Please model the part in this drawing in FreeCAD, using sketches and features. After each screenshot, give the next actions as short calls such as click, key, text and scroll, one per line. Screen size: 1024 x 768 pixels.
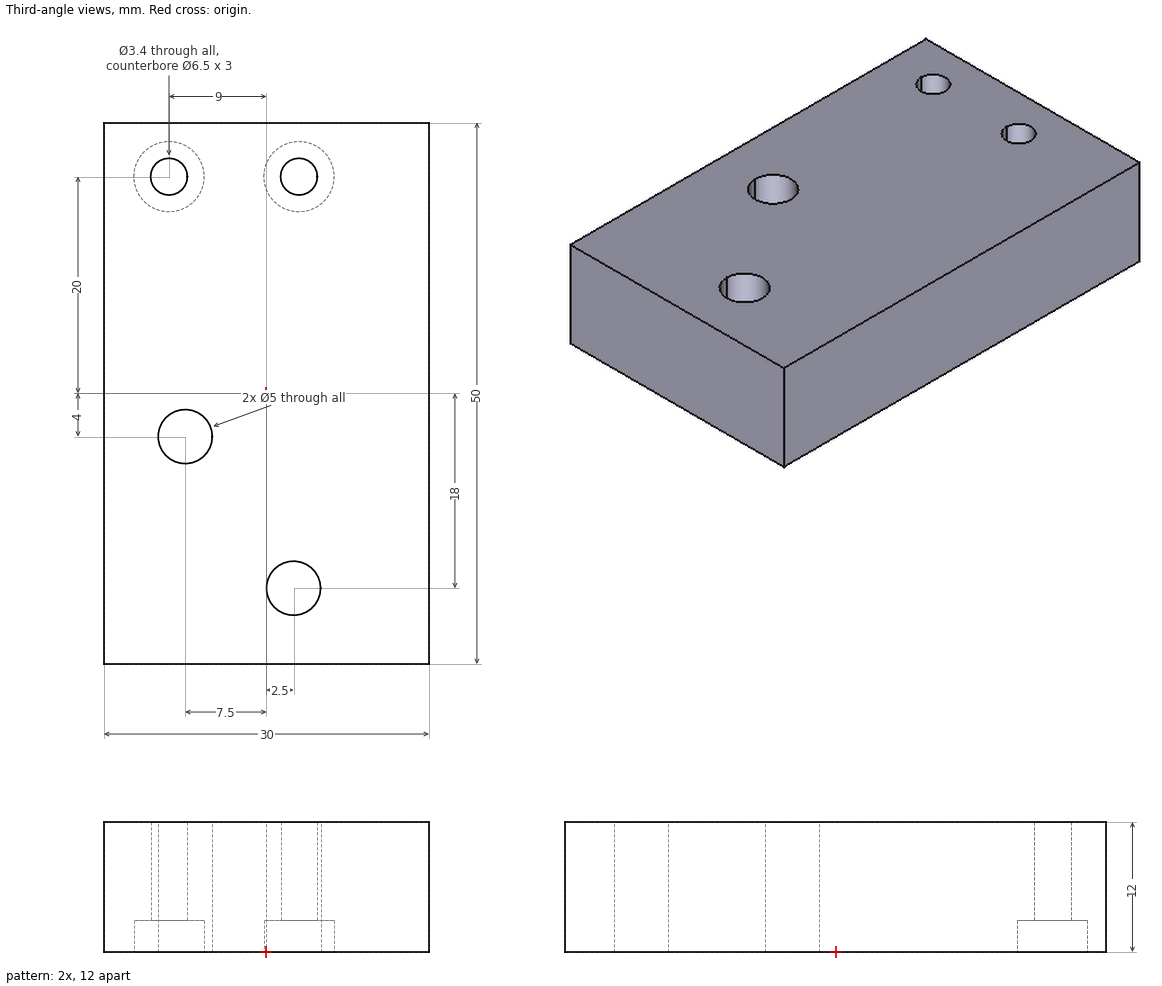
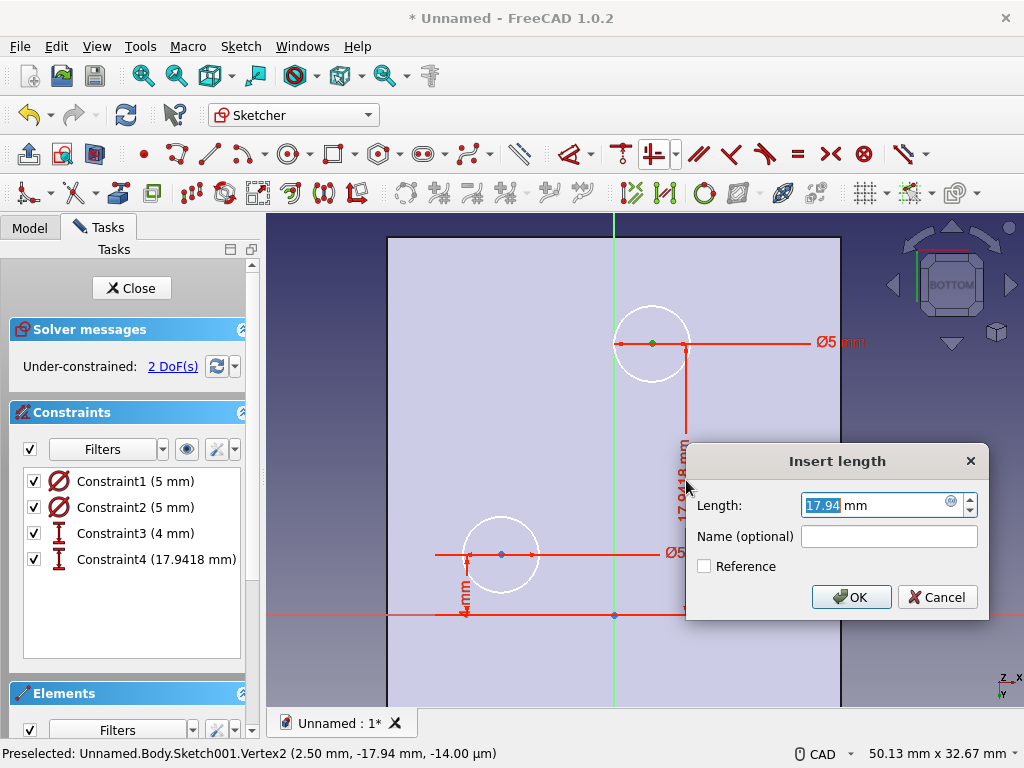
text(18)
key(Return)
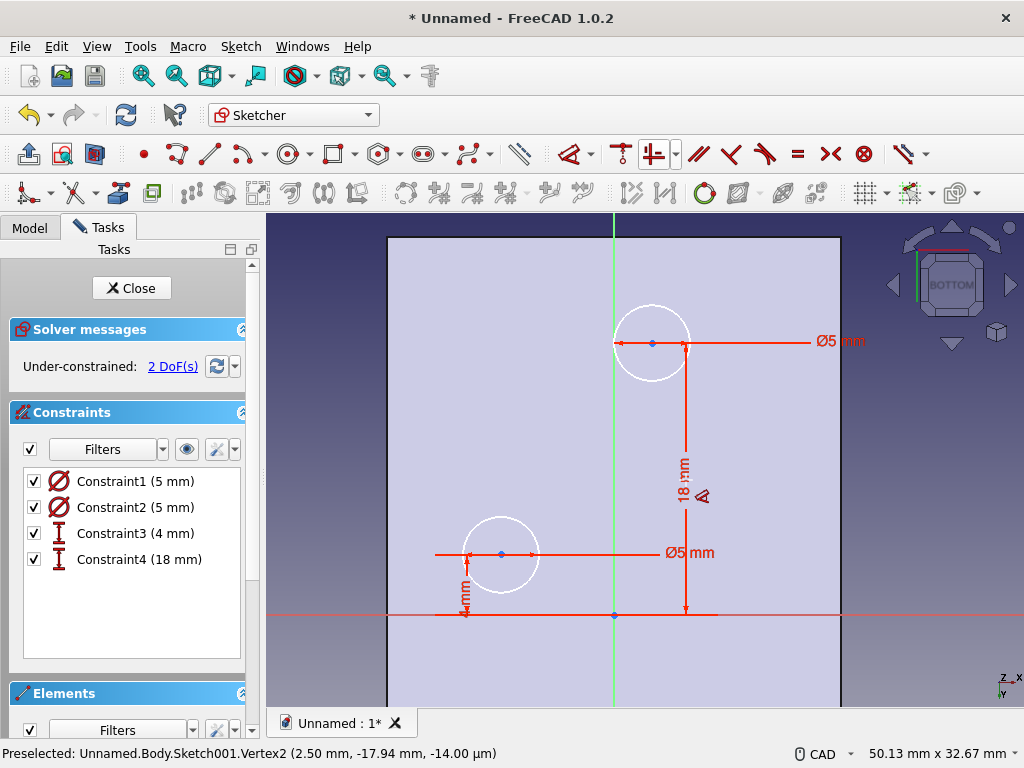
click(501, 555)
click(558, 649)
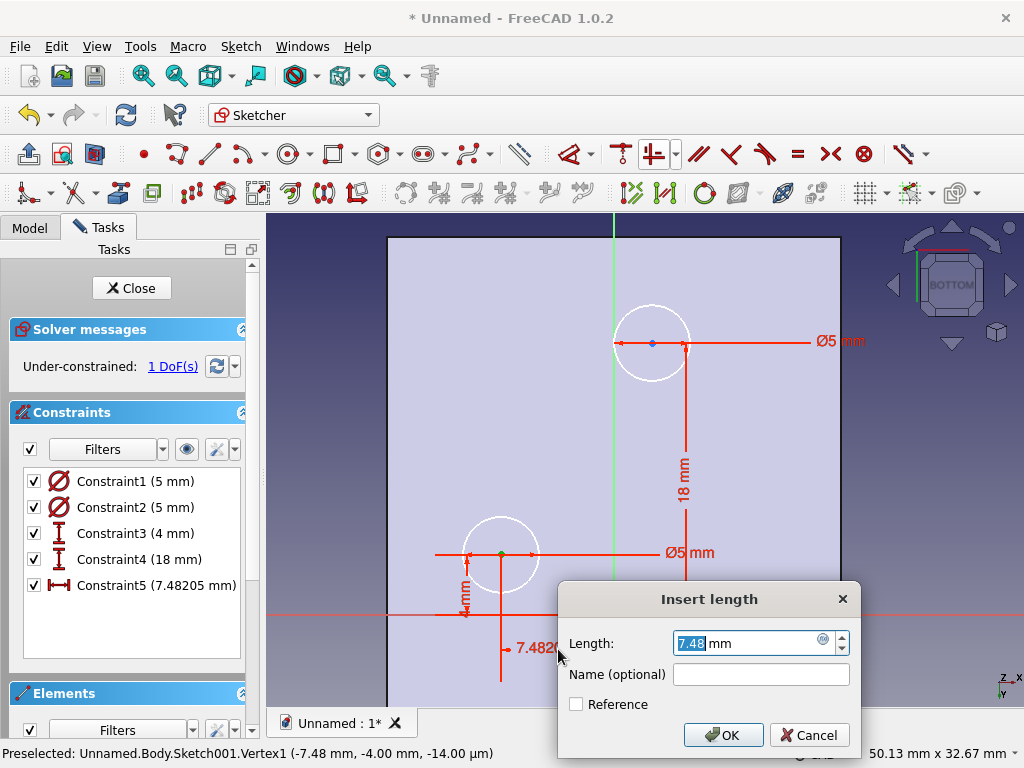
text(7.5)
key(Return)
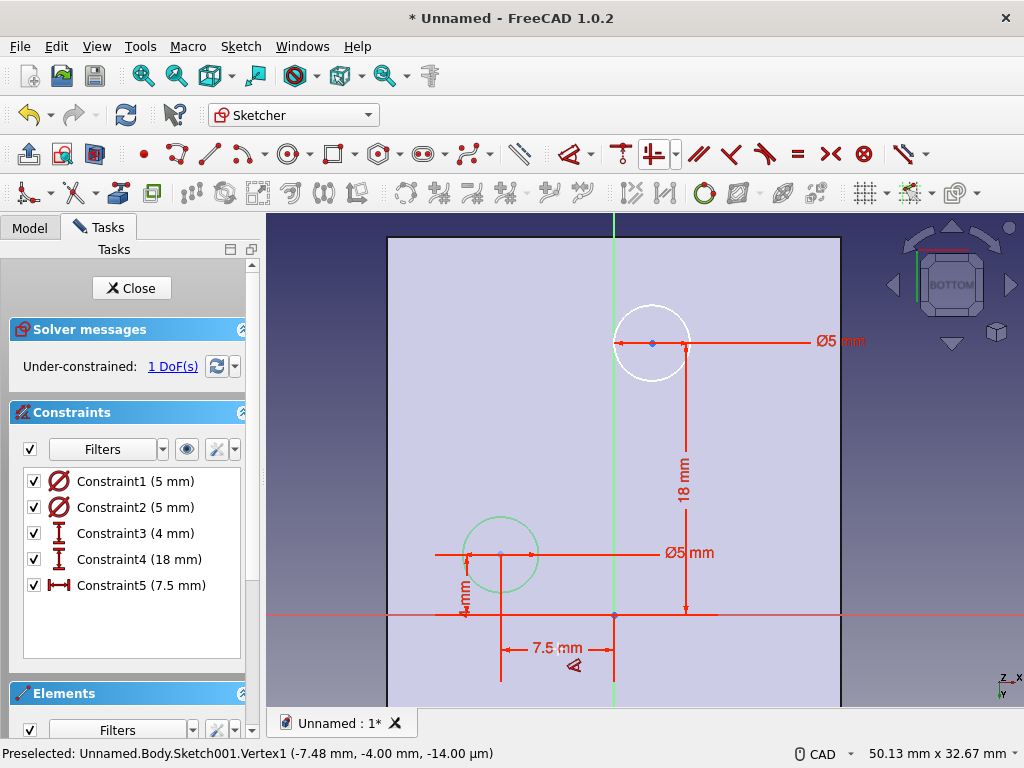
click(652, 343)
click(633, 649)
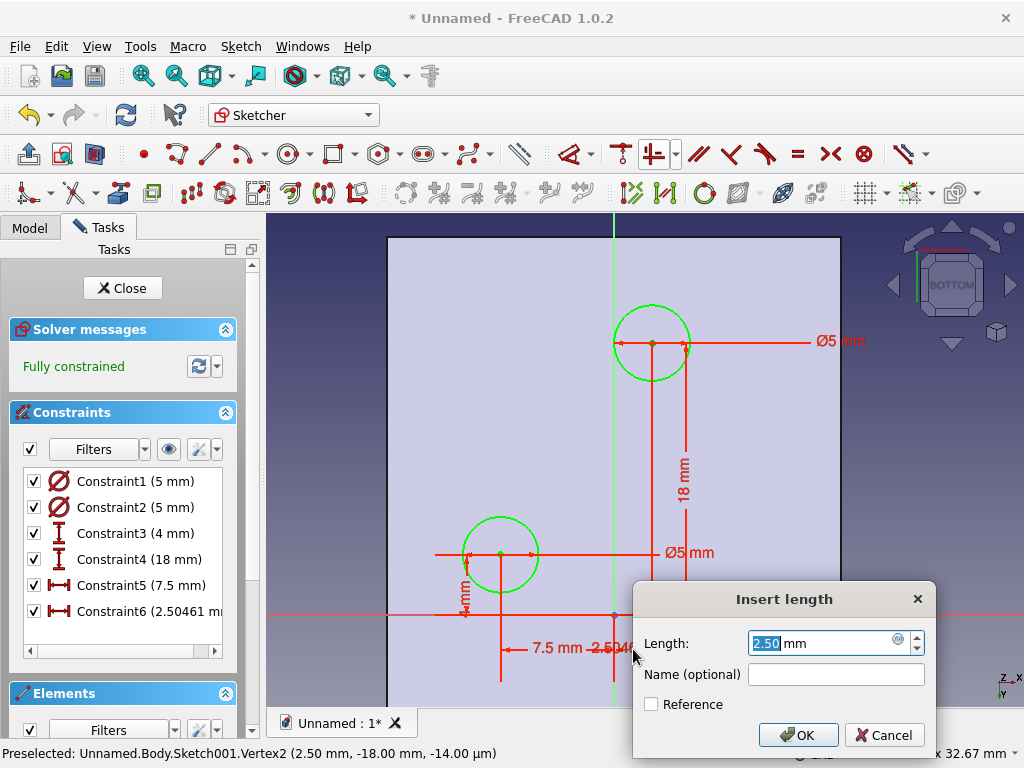
text(2.5)
key(Return)
key(Escape)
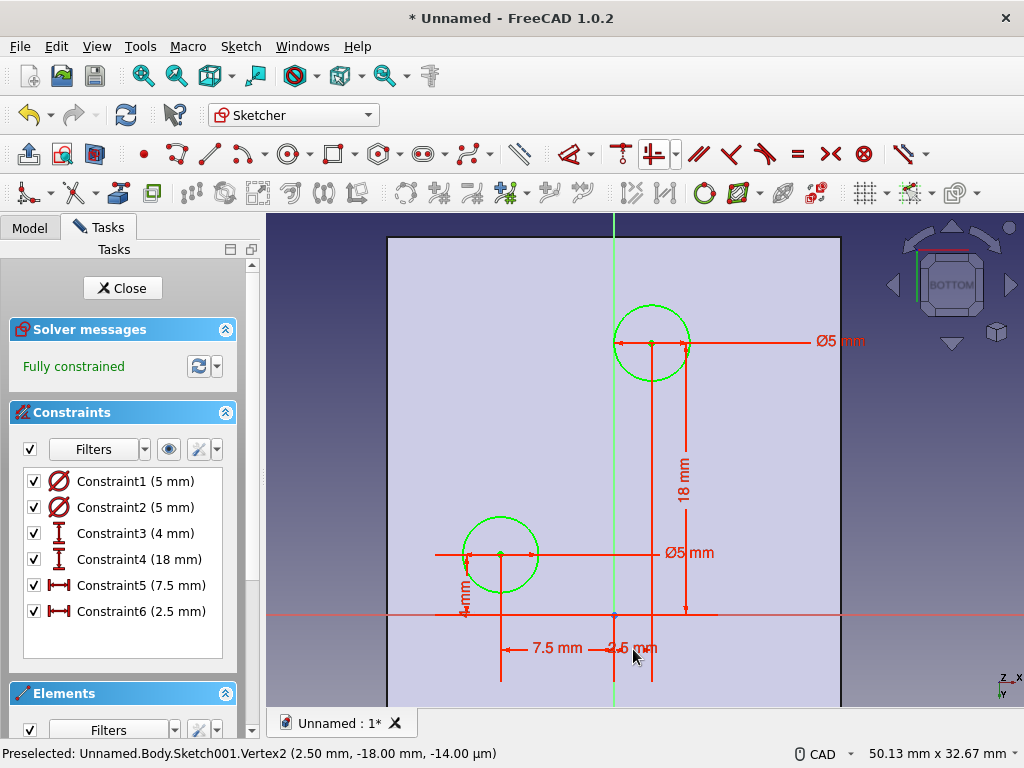
click(123, 288)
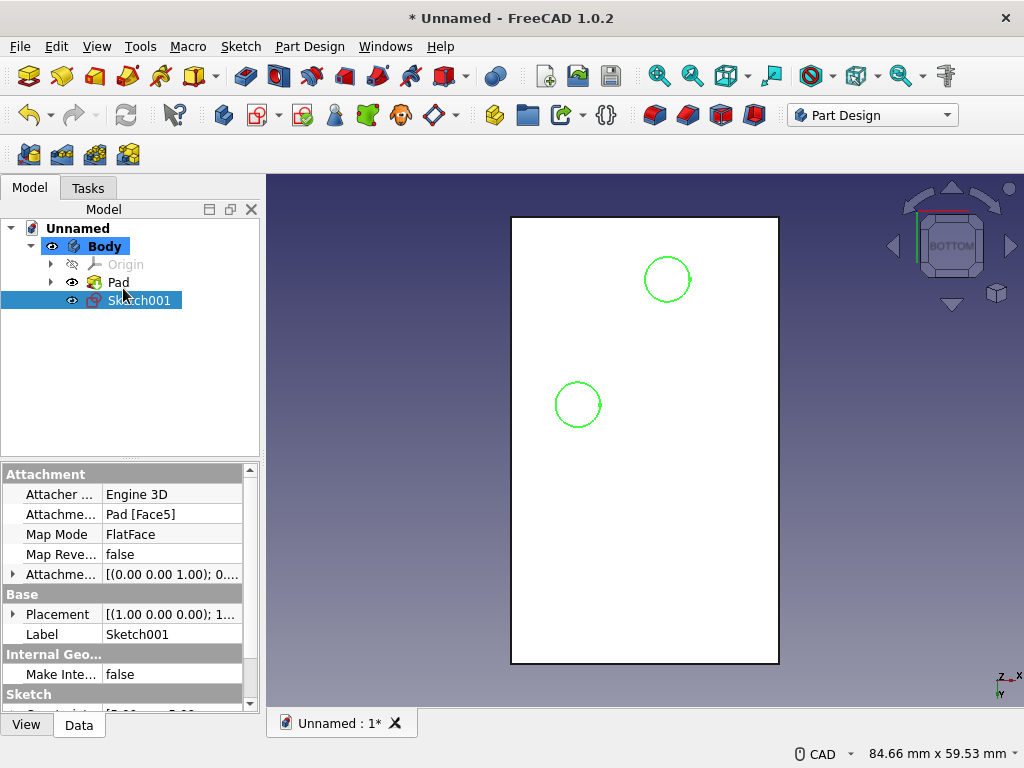
click(279, 76)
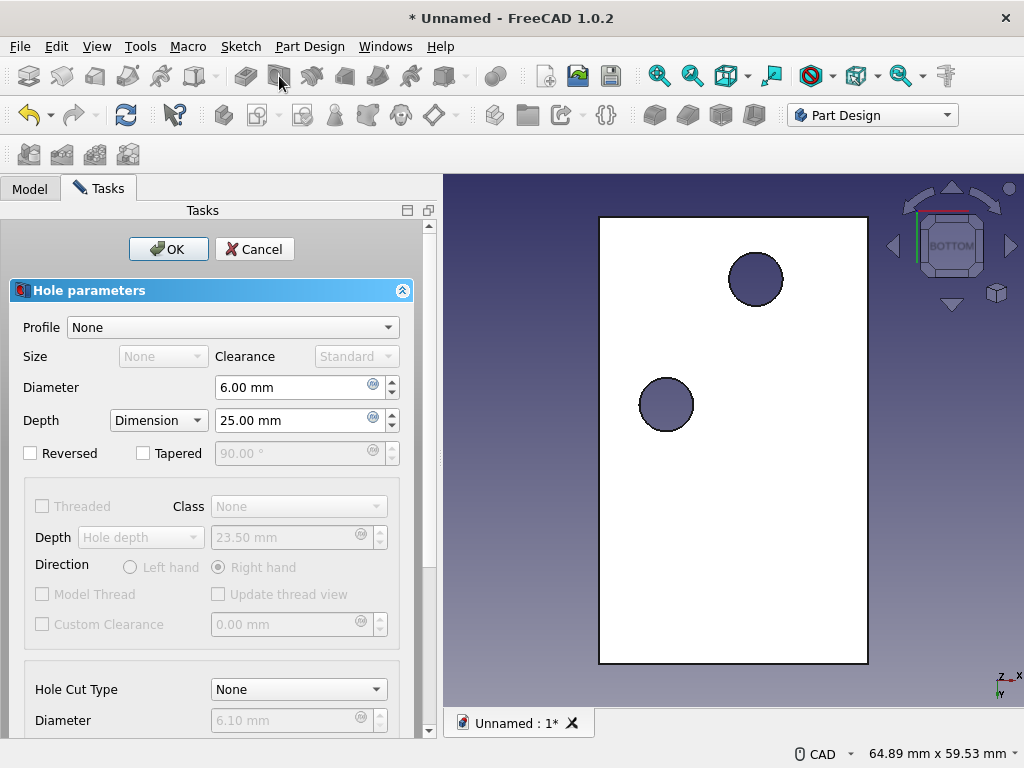
triple_click(300, 388)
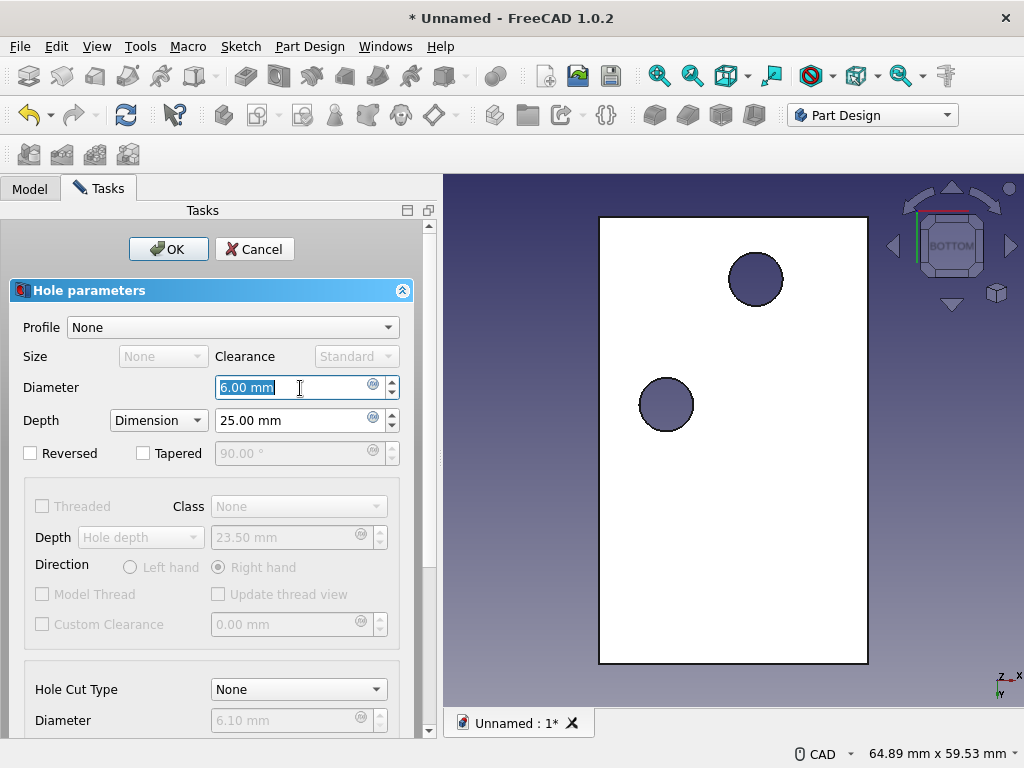
text(5)
key(Tab)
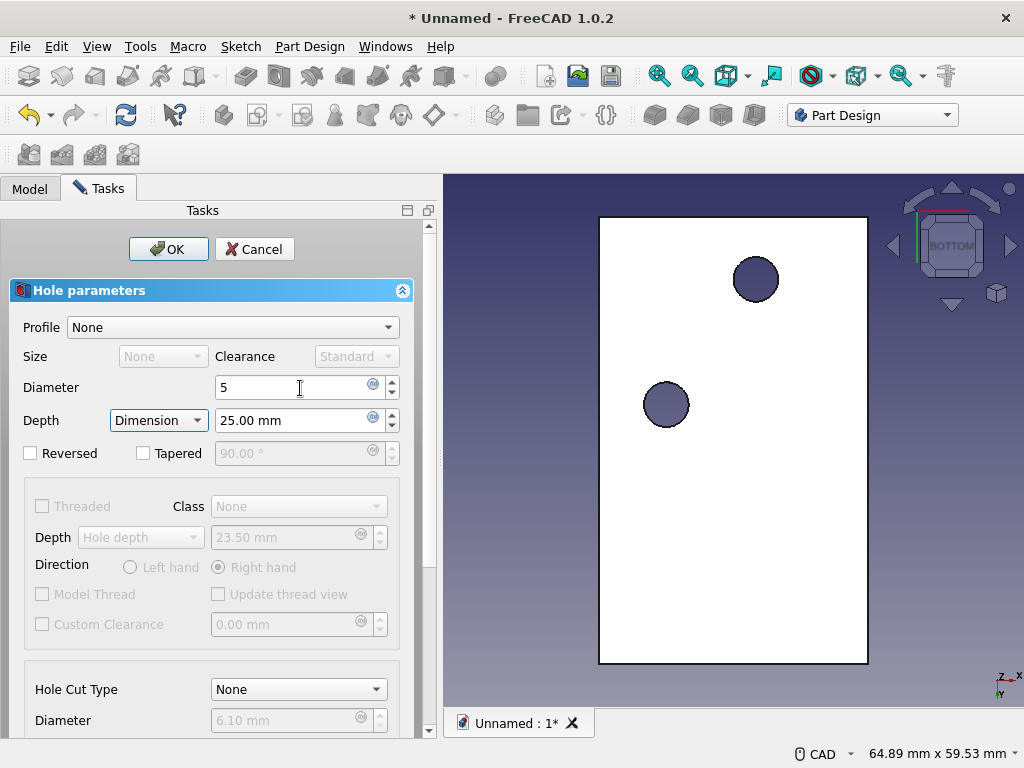
click(160, 420)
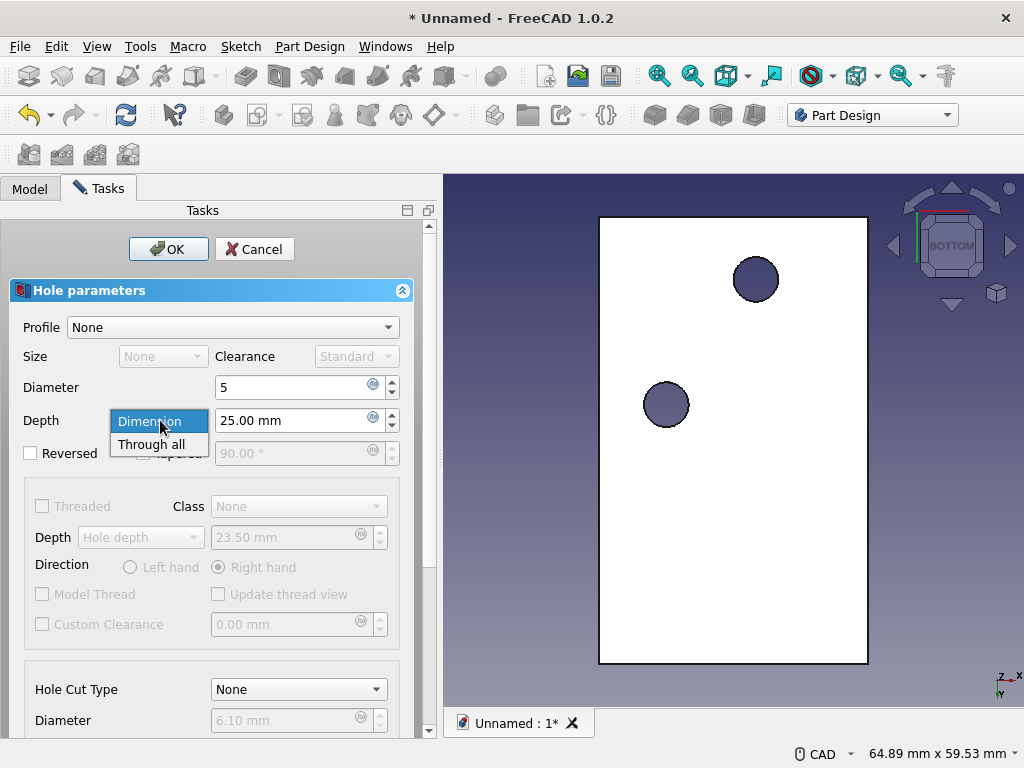
click(158, 444)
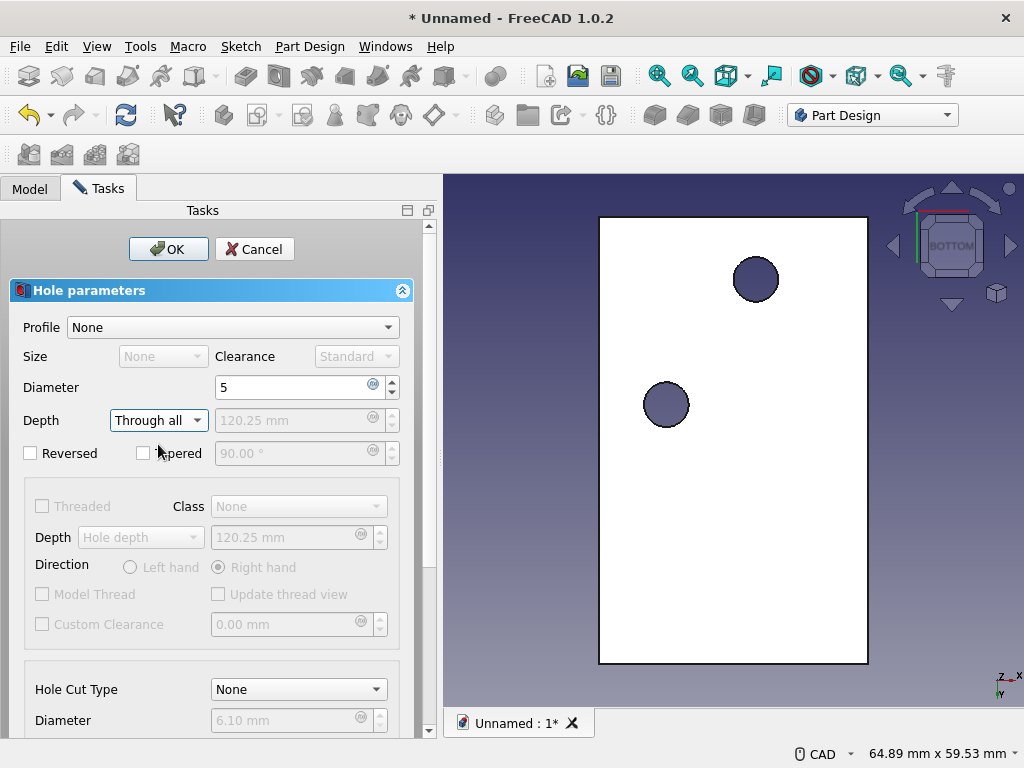
click(169, 249)